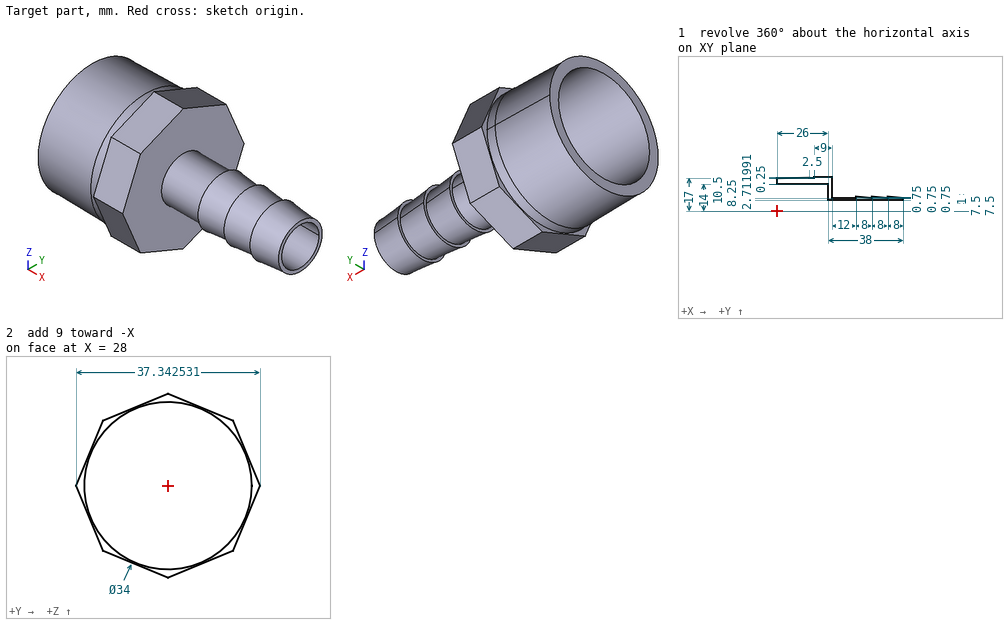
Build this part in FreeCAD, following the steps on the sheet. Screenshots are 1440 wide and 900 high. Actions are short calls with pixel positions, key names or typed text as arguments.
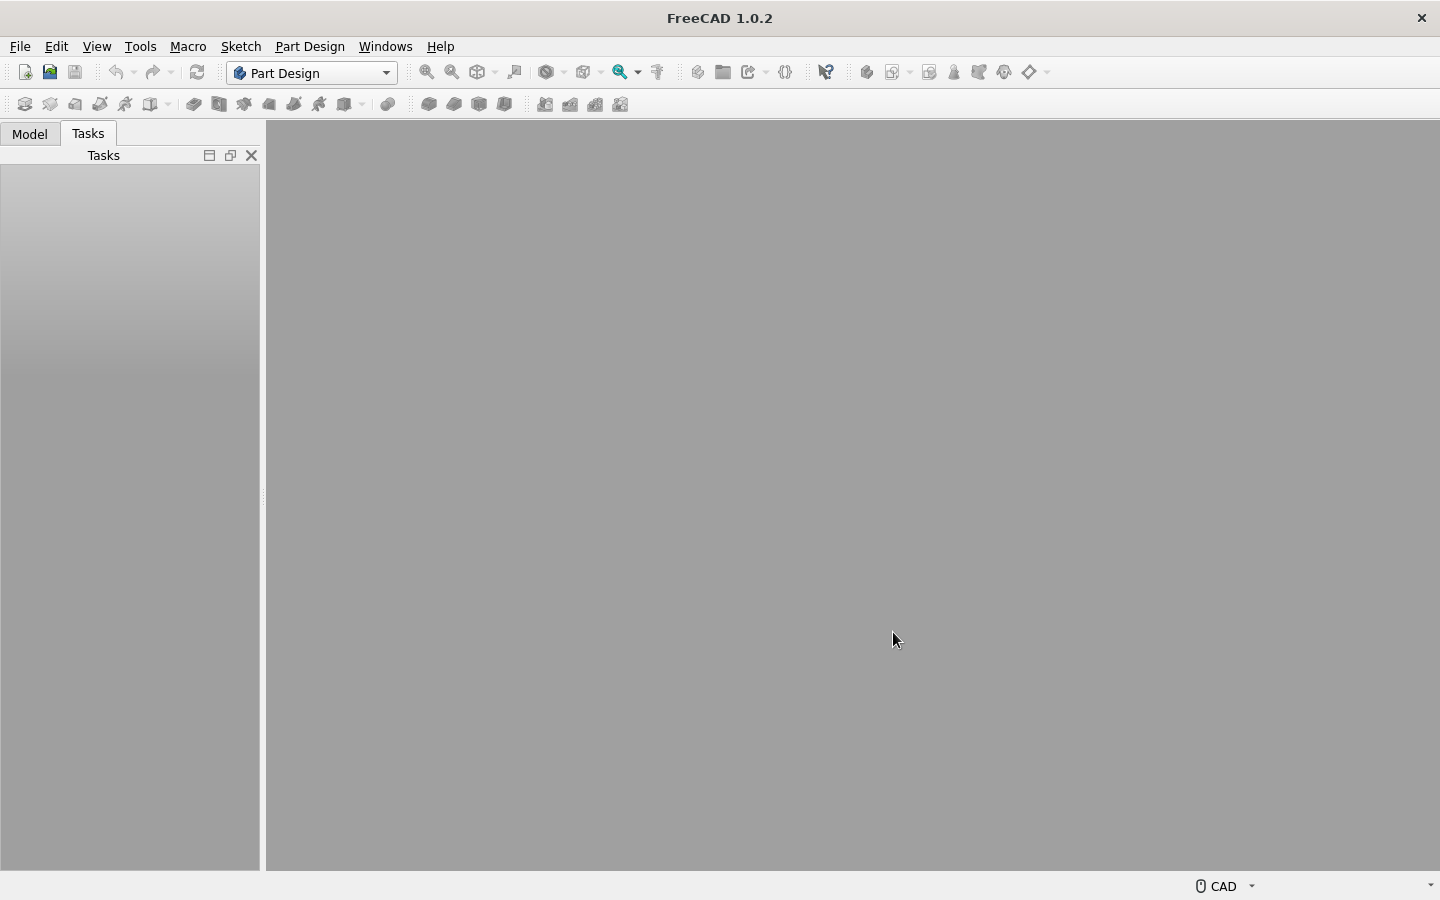
click(25, 72)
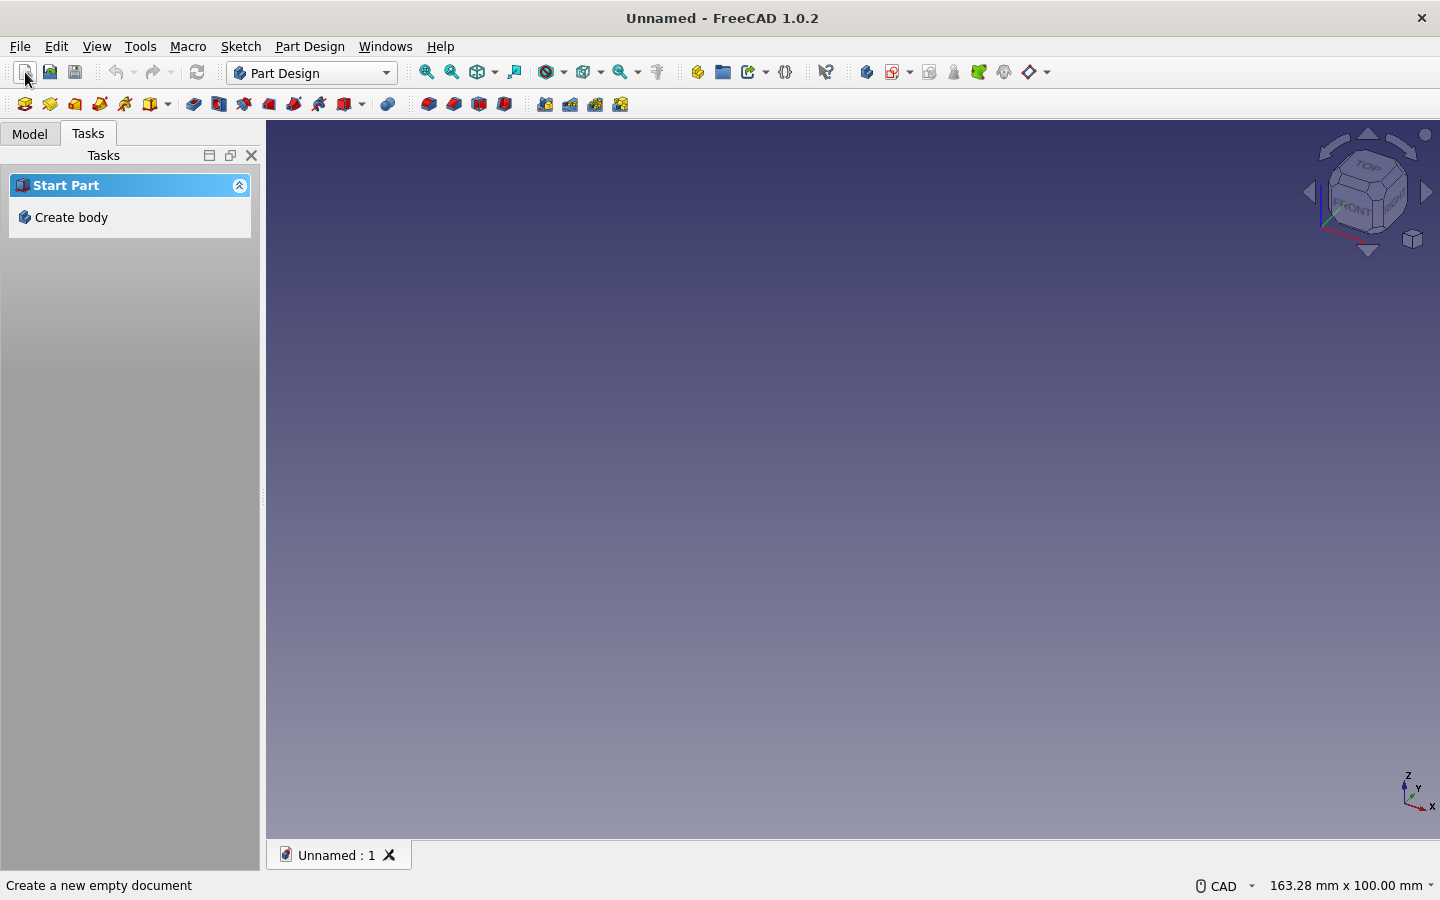
click(892, 72)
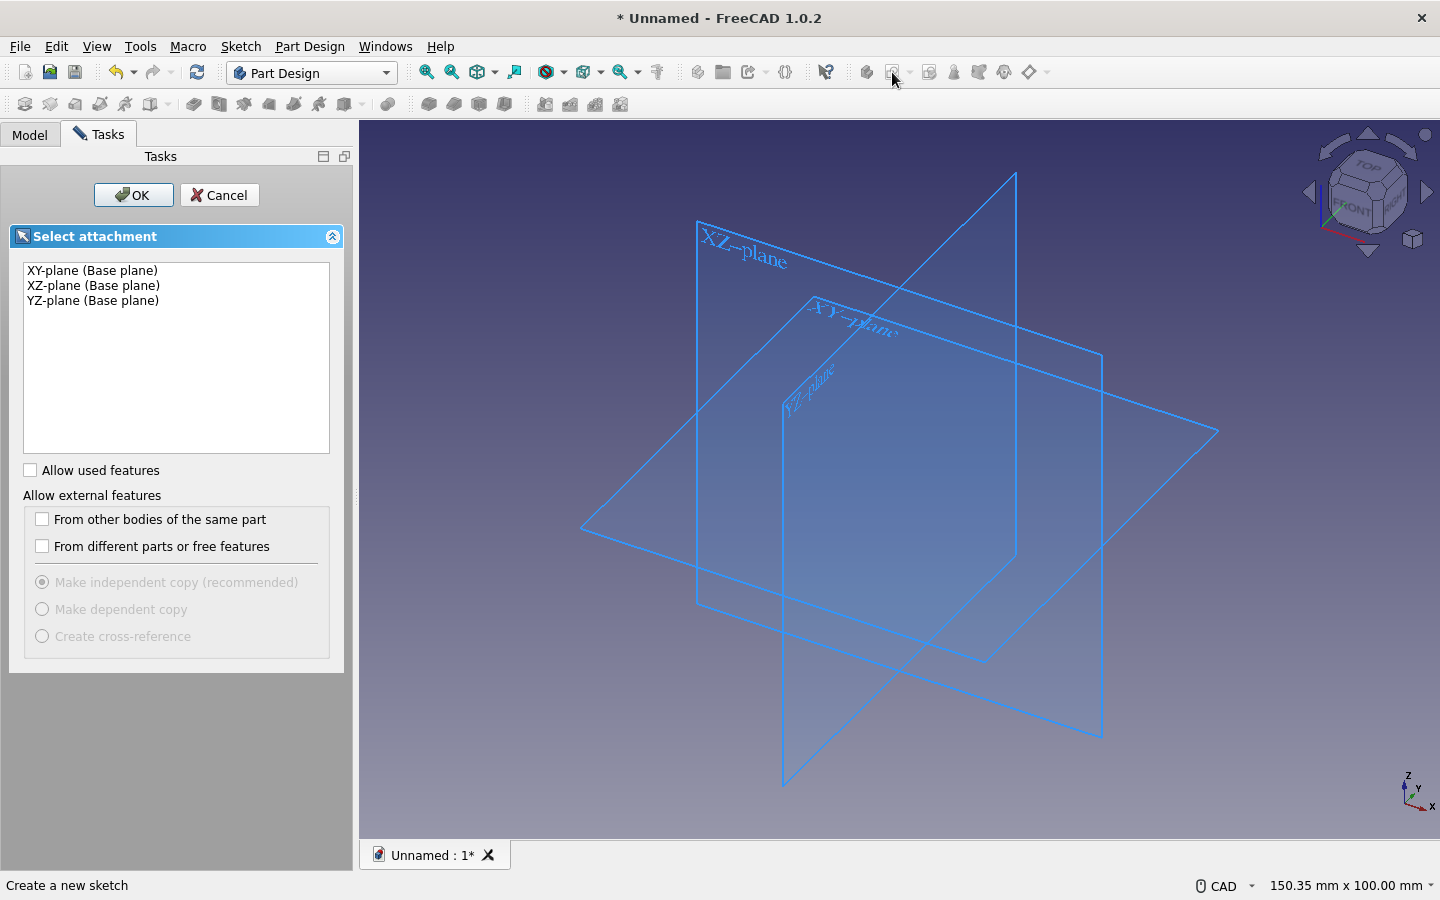
click(84, 270)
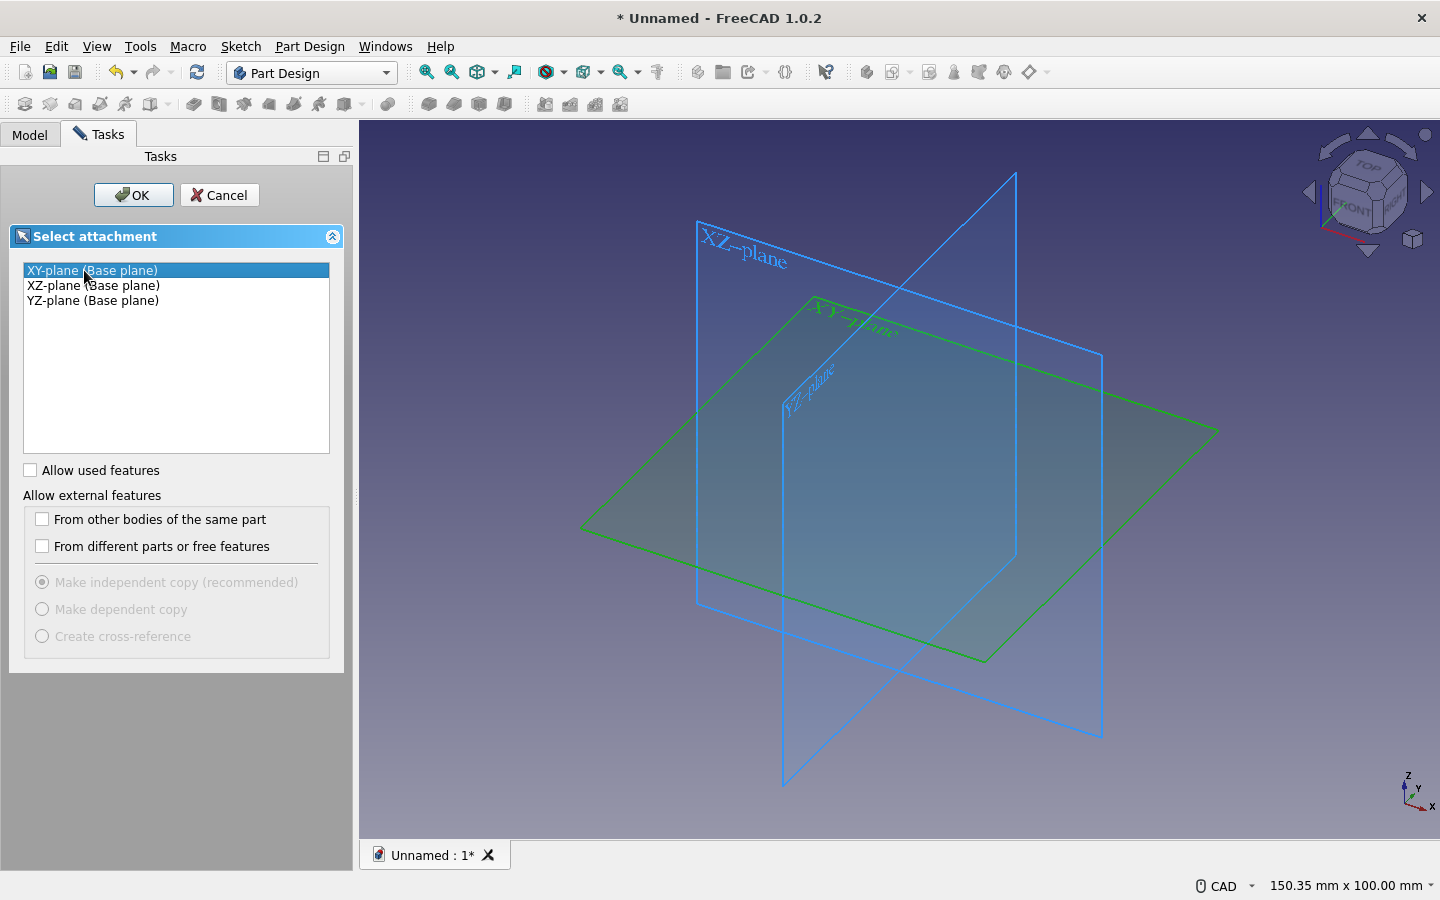
click(134, 195)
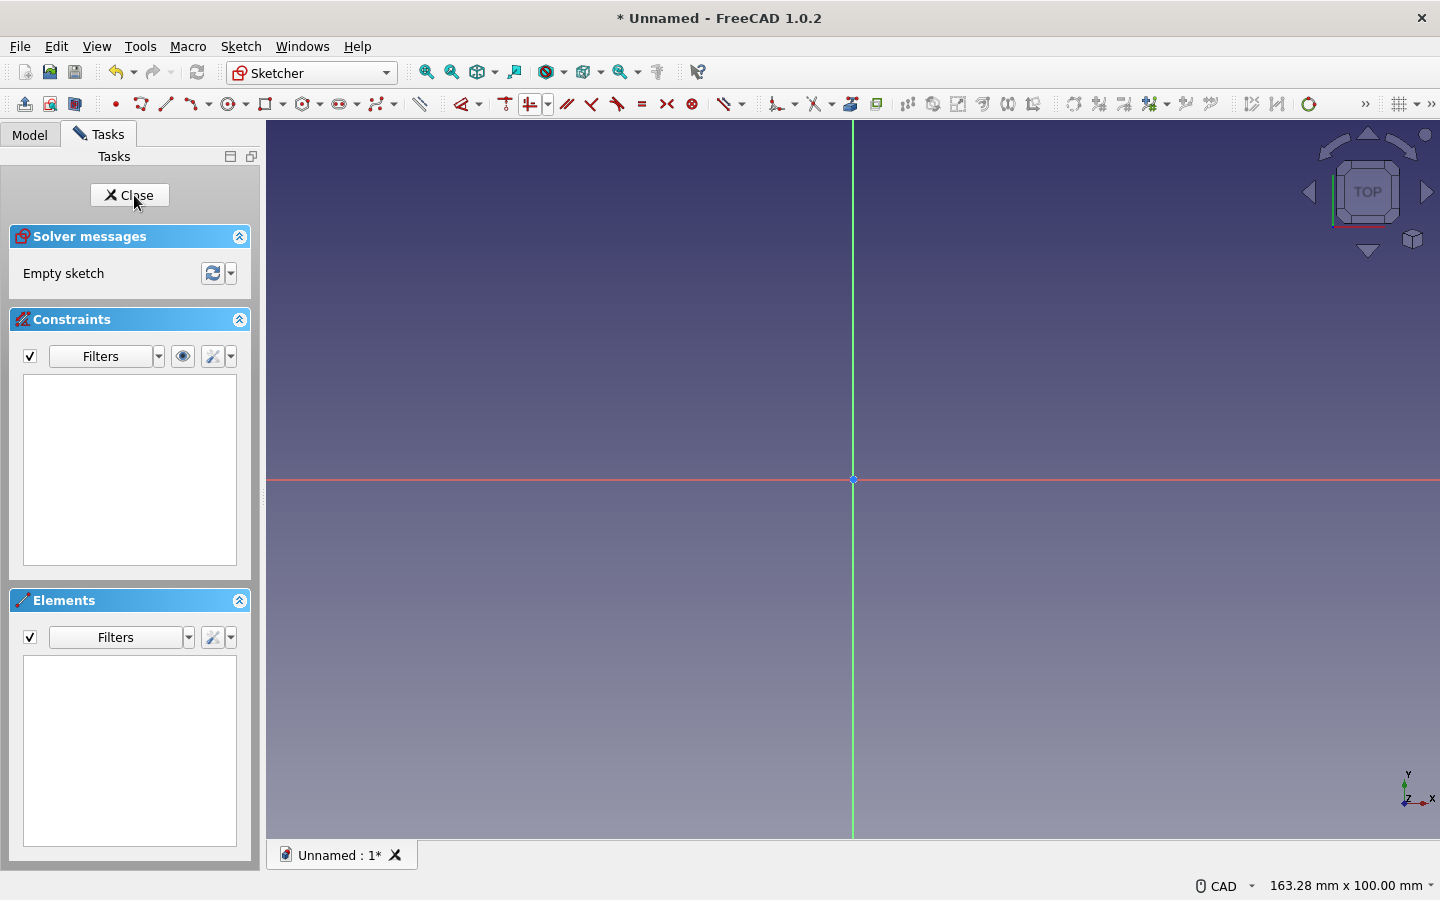
scroll(294, 760, down, 1)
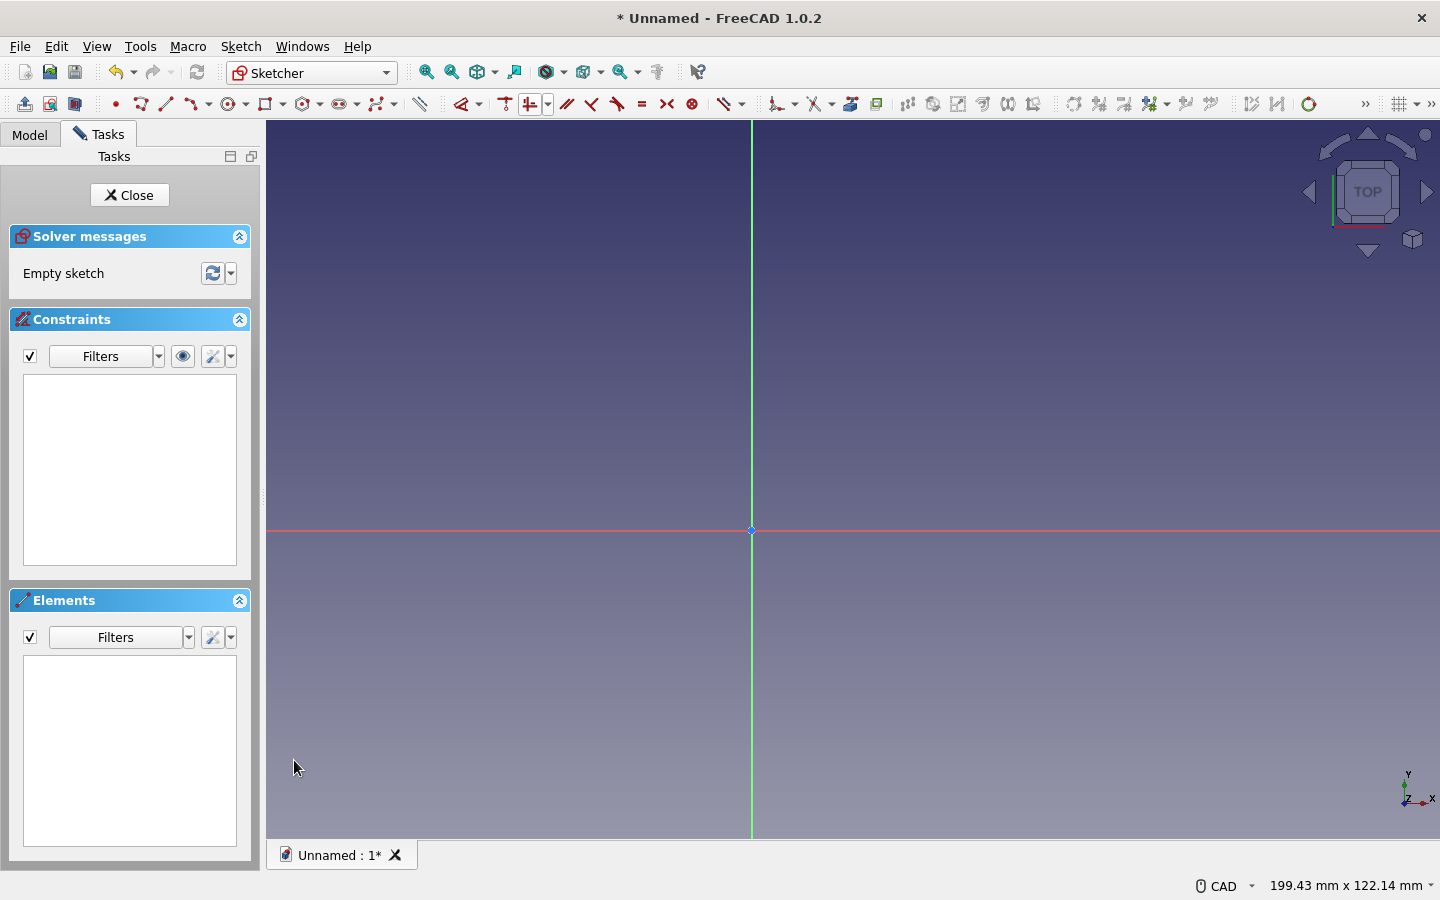
scroll(1129, 480, up, 3)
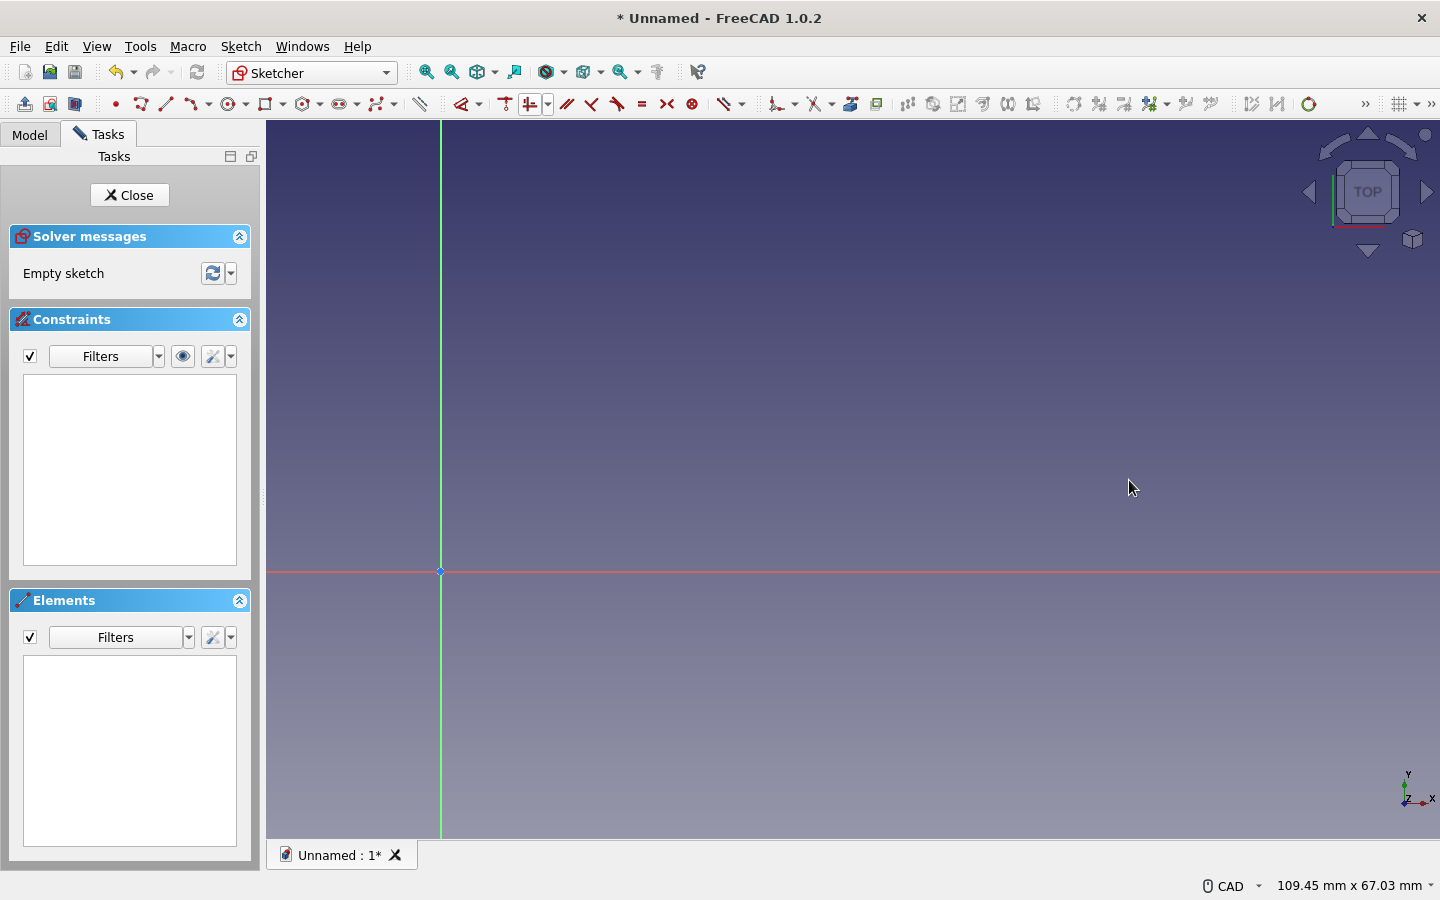
click(141, 104)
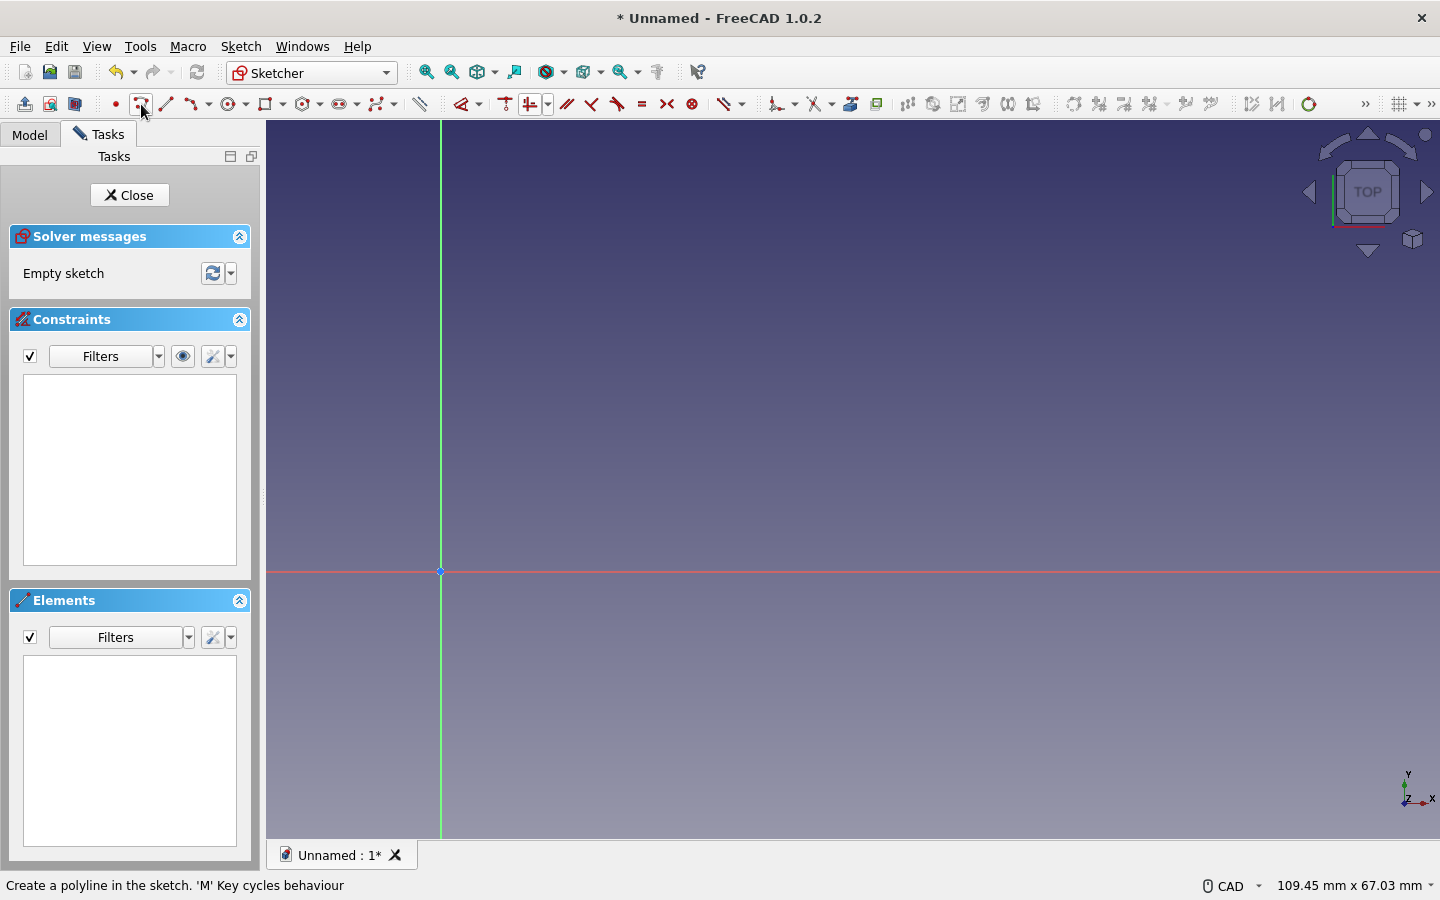
click(441, 421)
click(720, 421)
click(720, 510)
click(1127, 510)